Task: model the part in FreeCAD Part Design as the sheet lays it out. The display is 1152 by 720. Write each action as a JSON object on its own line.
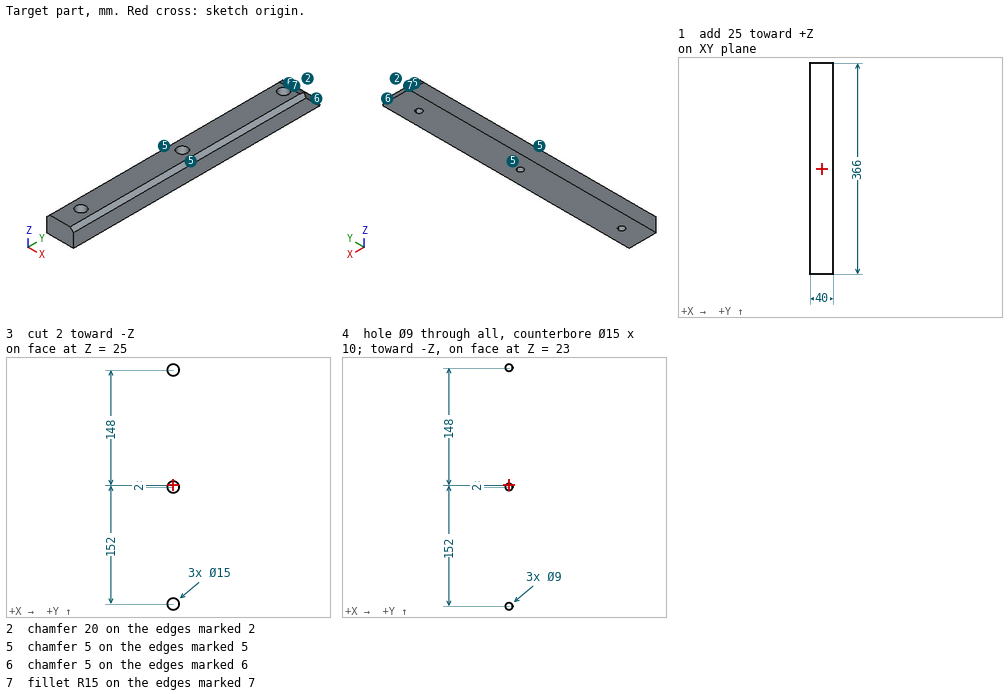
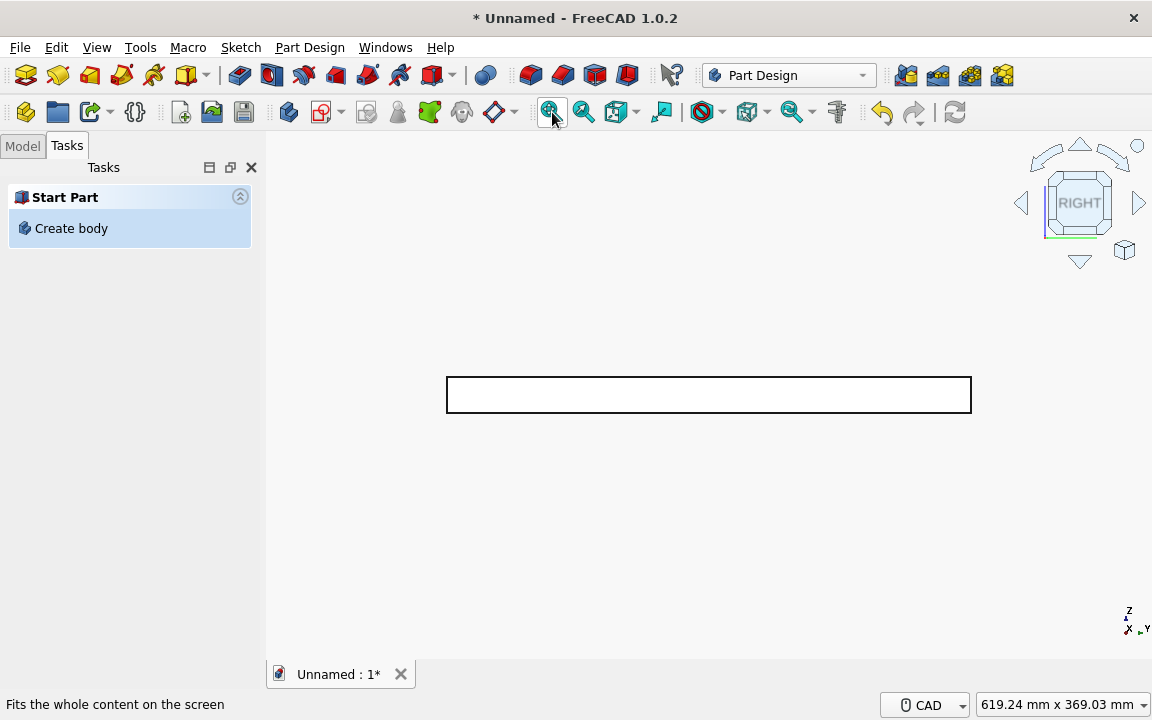
{"action": "key", "text": "5"}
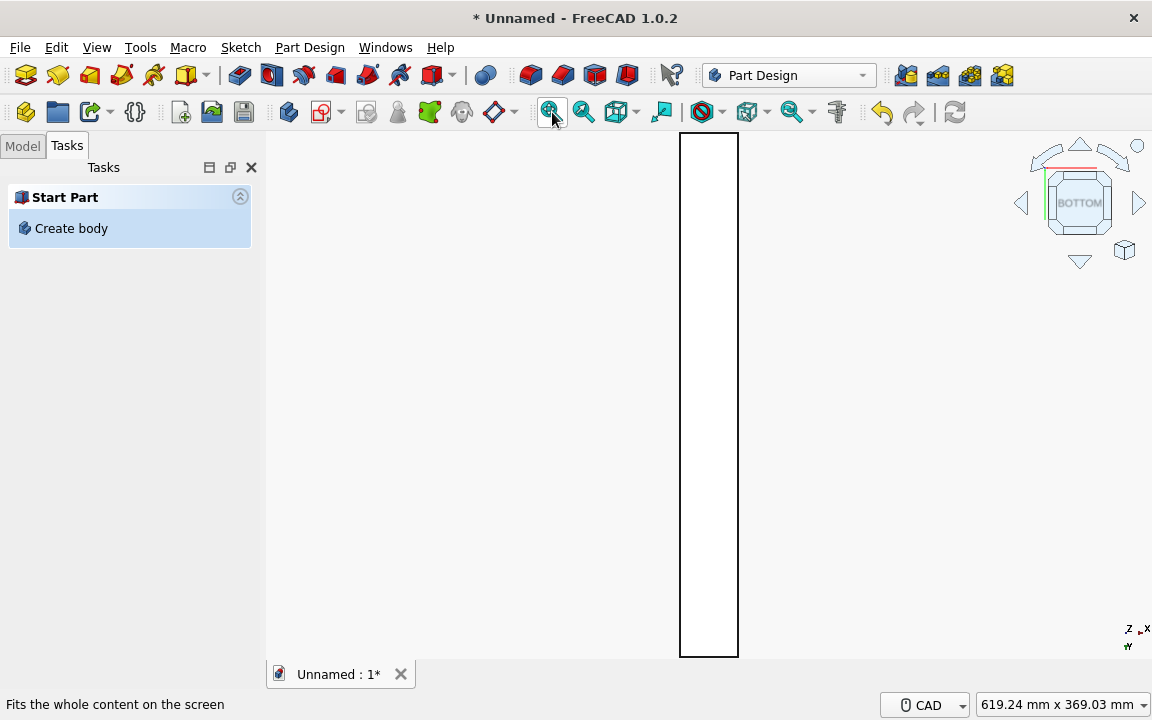
{"action": "key", "text": "4"}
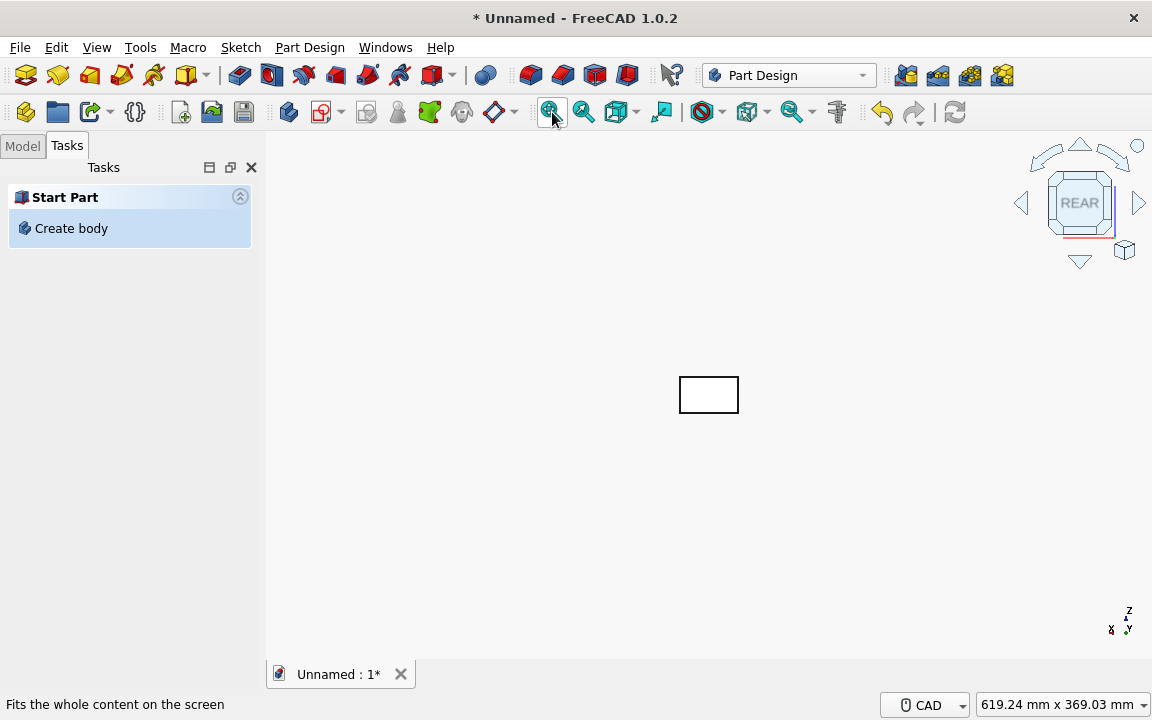
{"action": "left_click", "coordinate": [552, 112]}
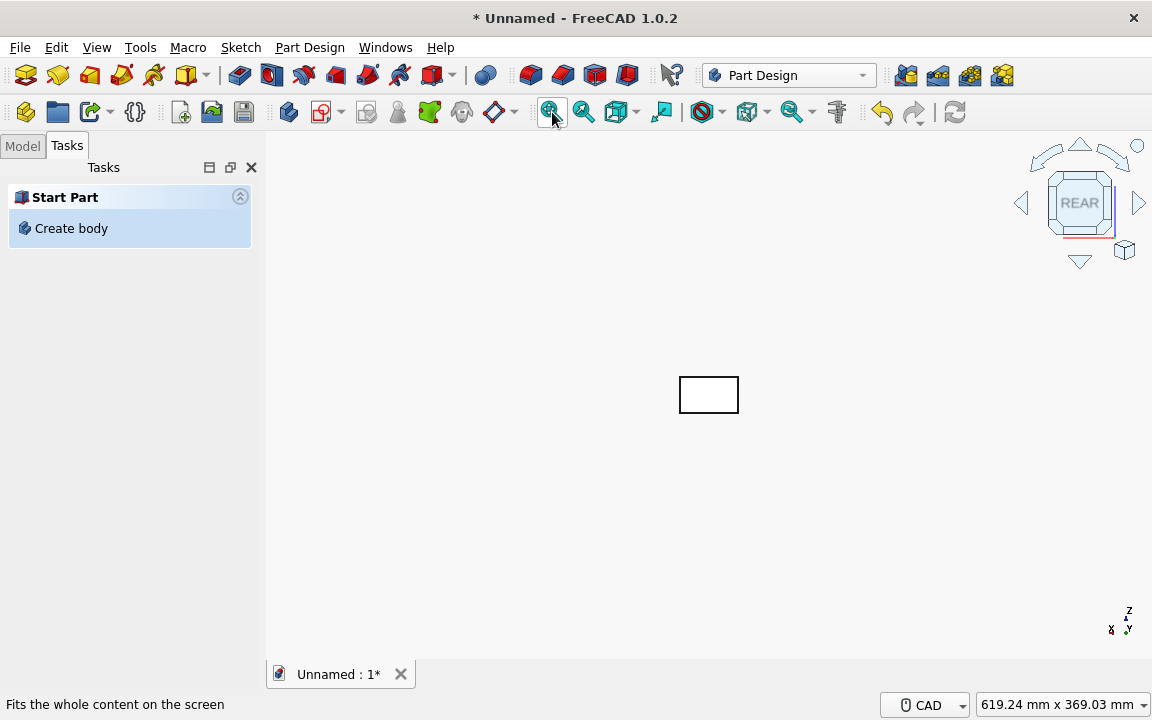
{"action": "left_click", "coordinate": [709, 376]}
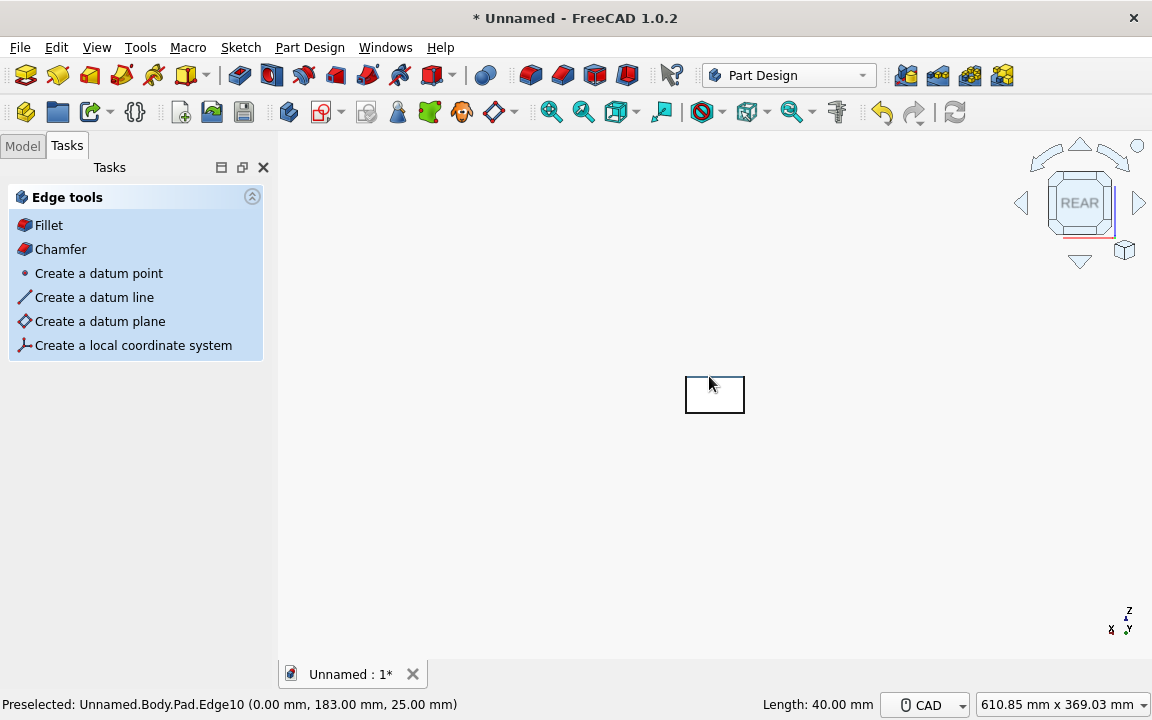
{"action": "left_click", "coordinate": [564, 76]}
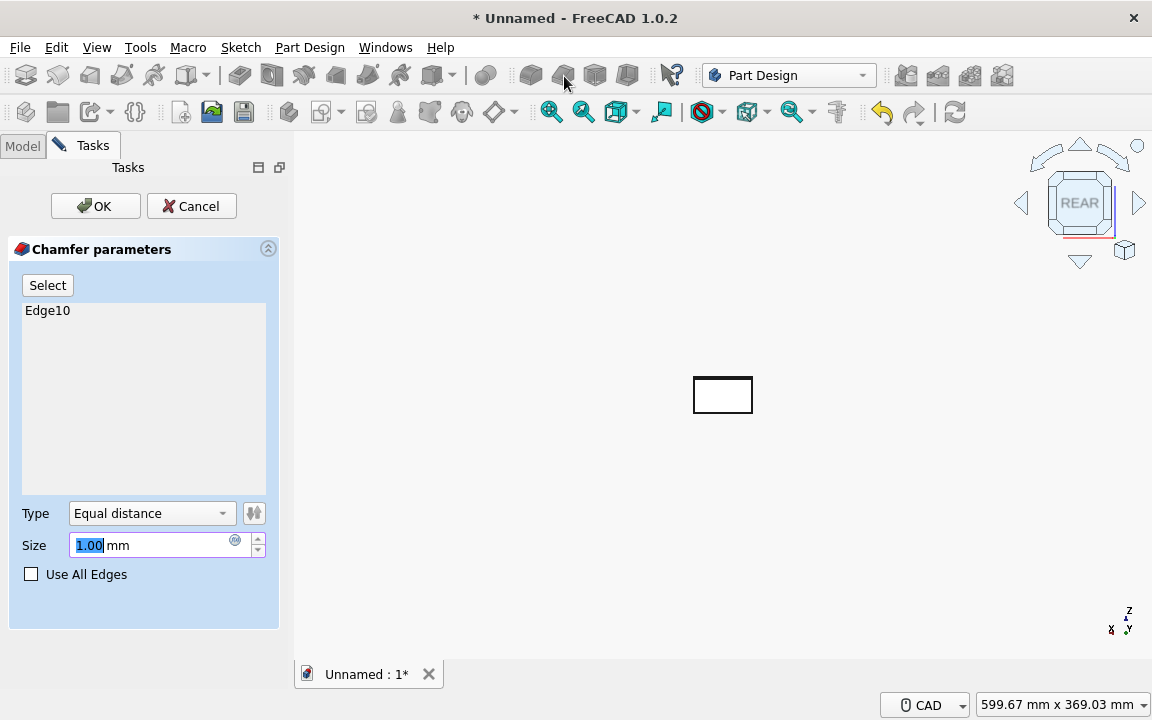
{"action": "type", "text": "20"}
{"action": "key", "text": "Tab"}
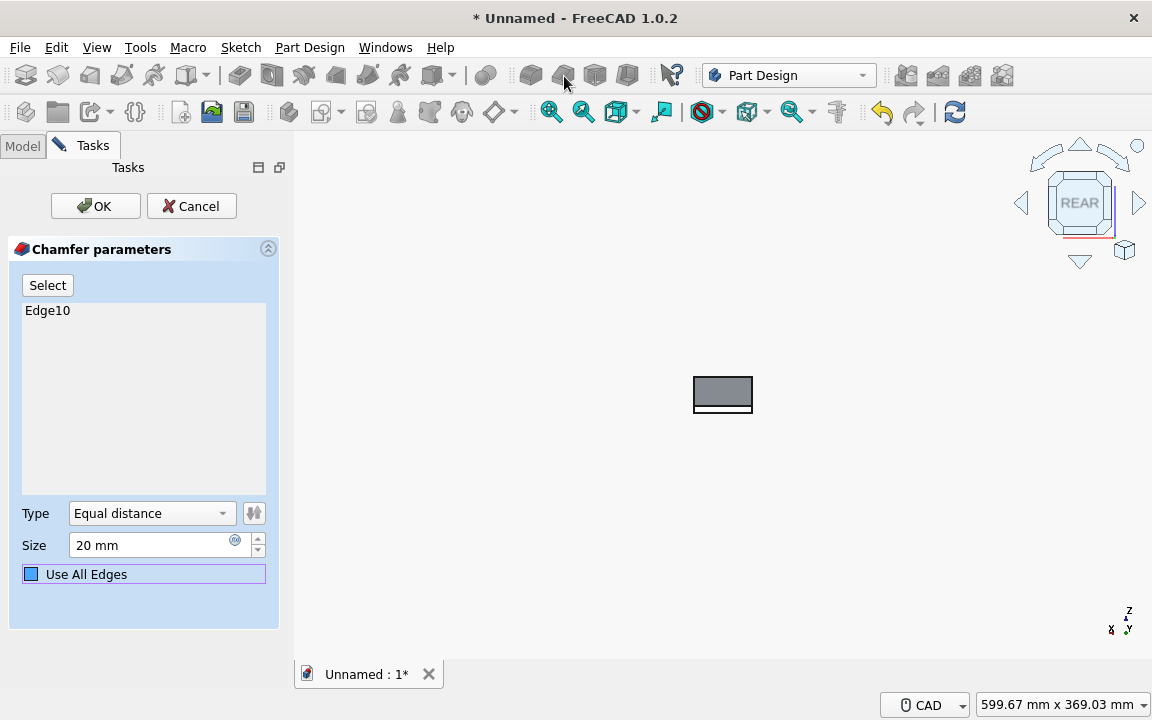
{"action": "left_click", "coordinate": [96, 206]}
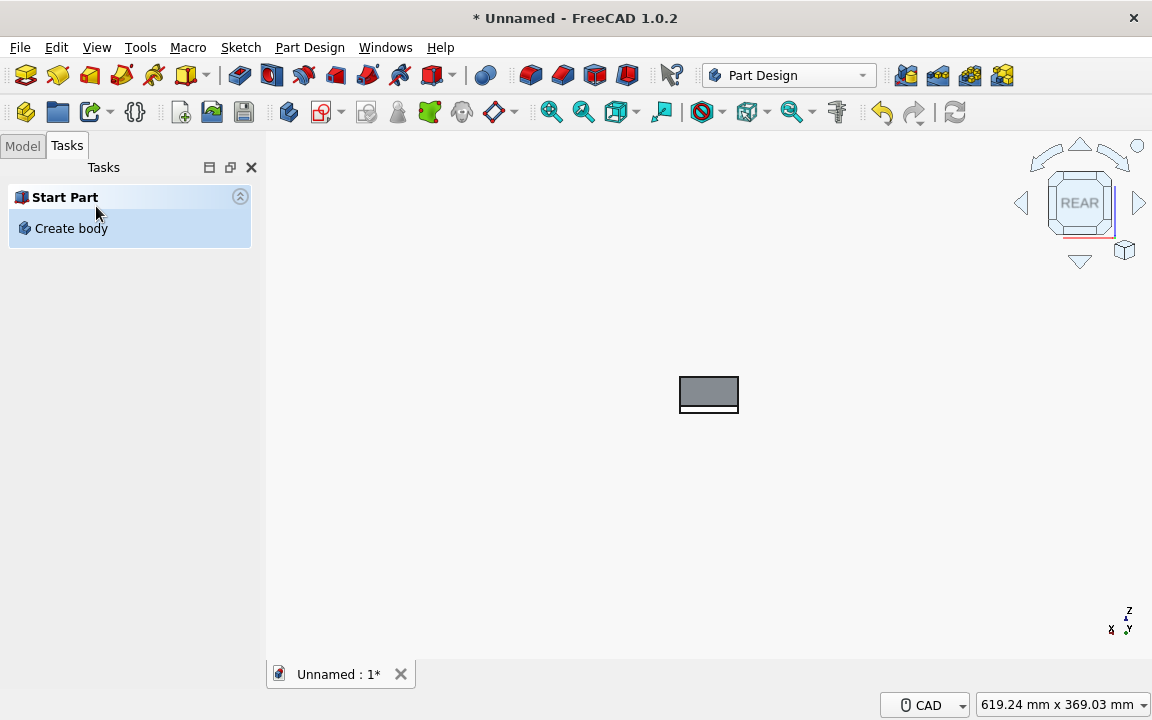
{"action": "key", "text": "v f"}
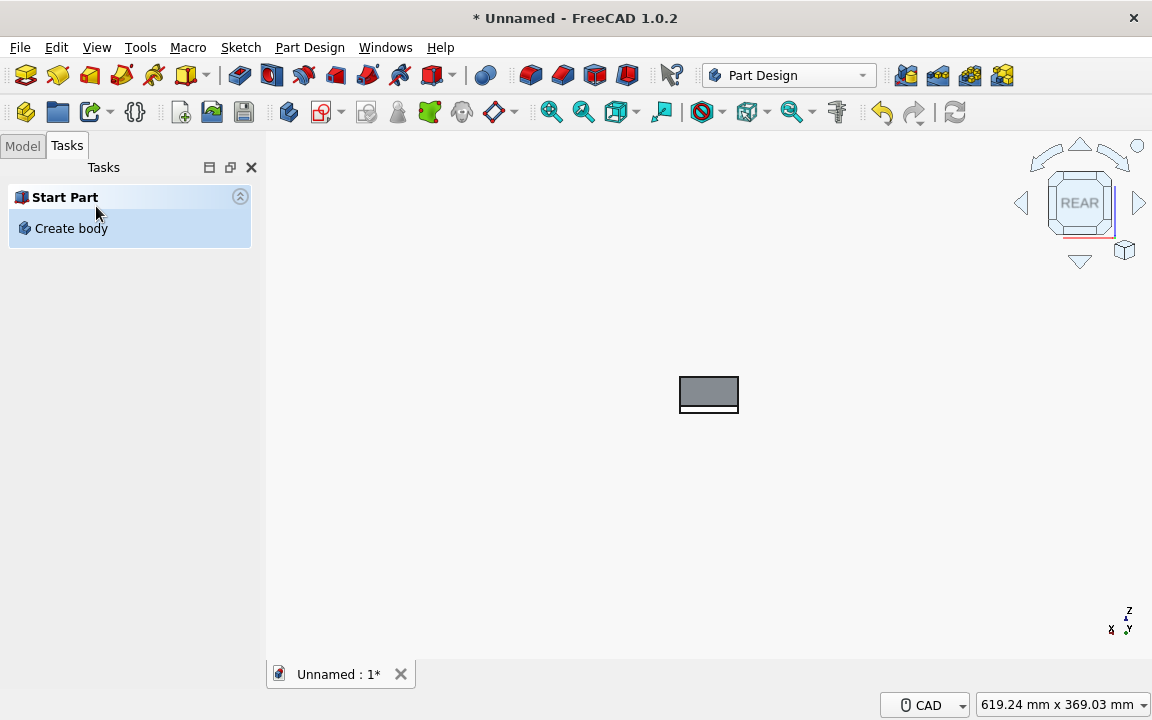
{"action": "key", "text": "0"}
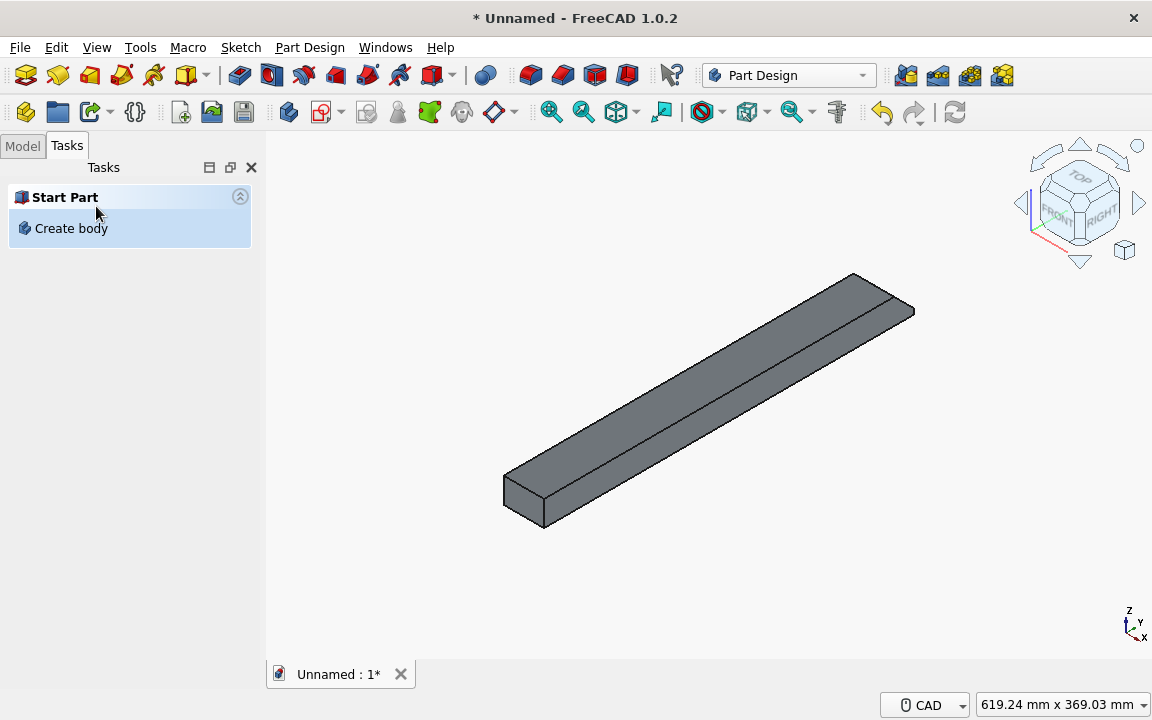
{"action": "left_click", "coordinate": [849, 299]}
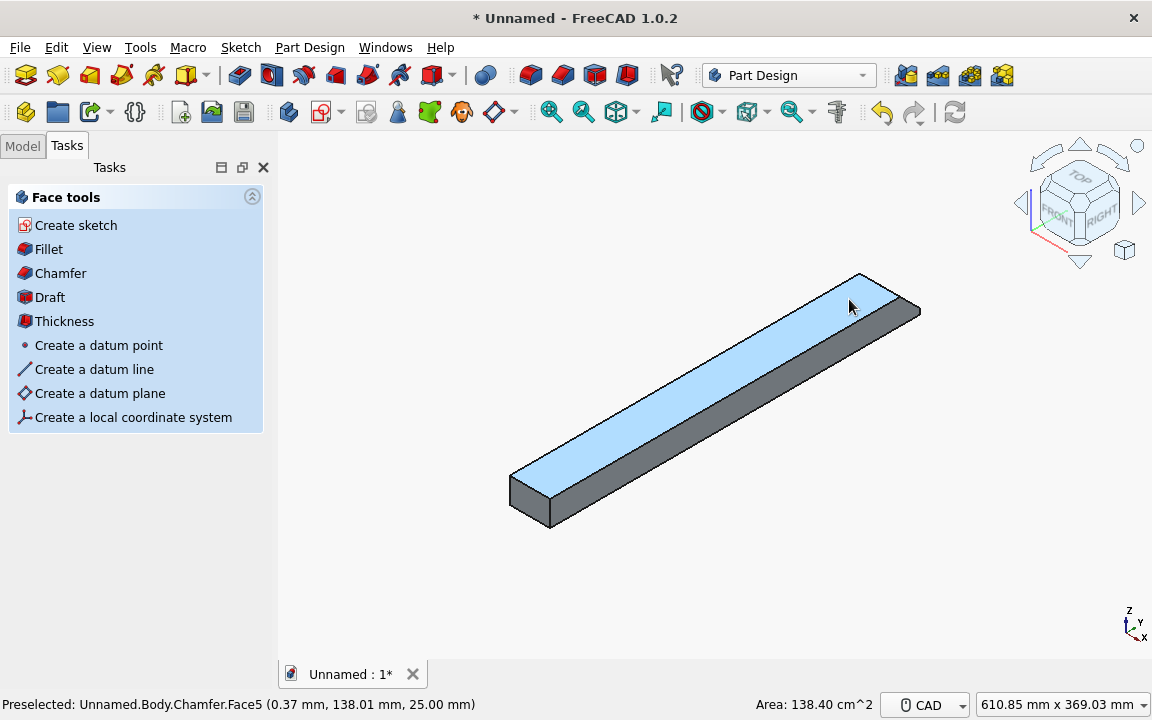
{"action": "left_click", "coordinate": [322, 112]}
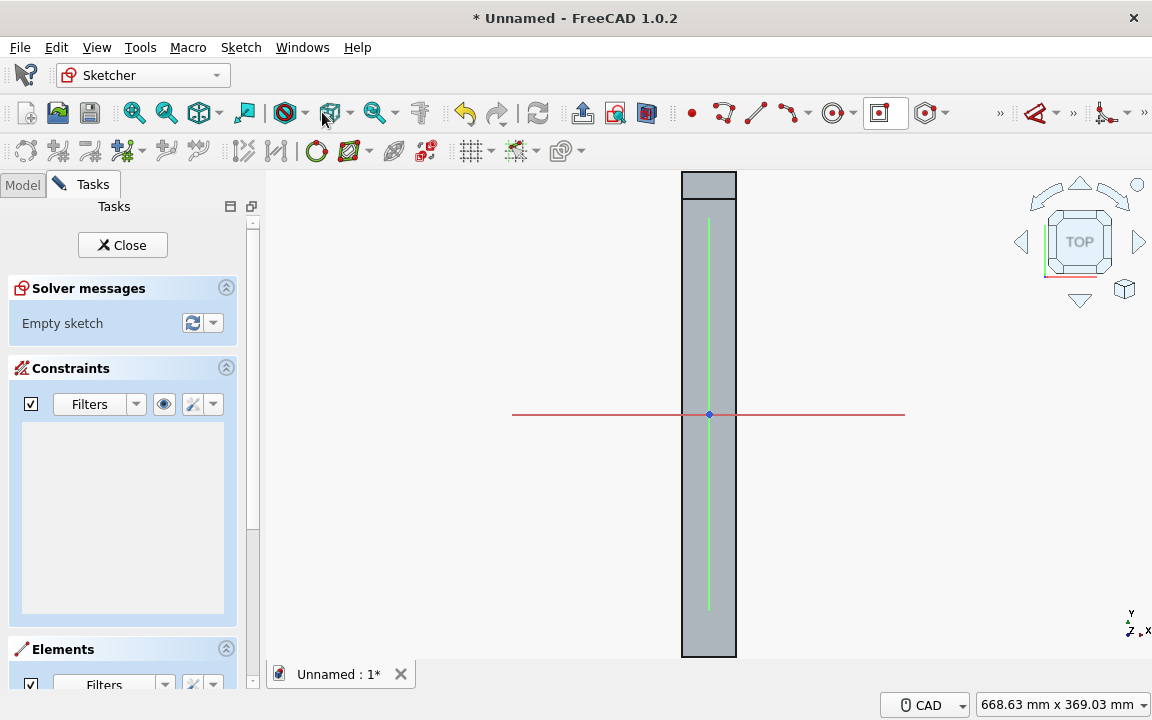
{"action": "scroll", "coordinate": [501, 409], "scroll_direction": "down", "scroll_amount": 2}